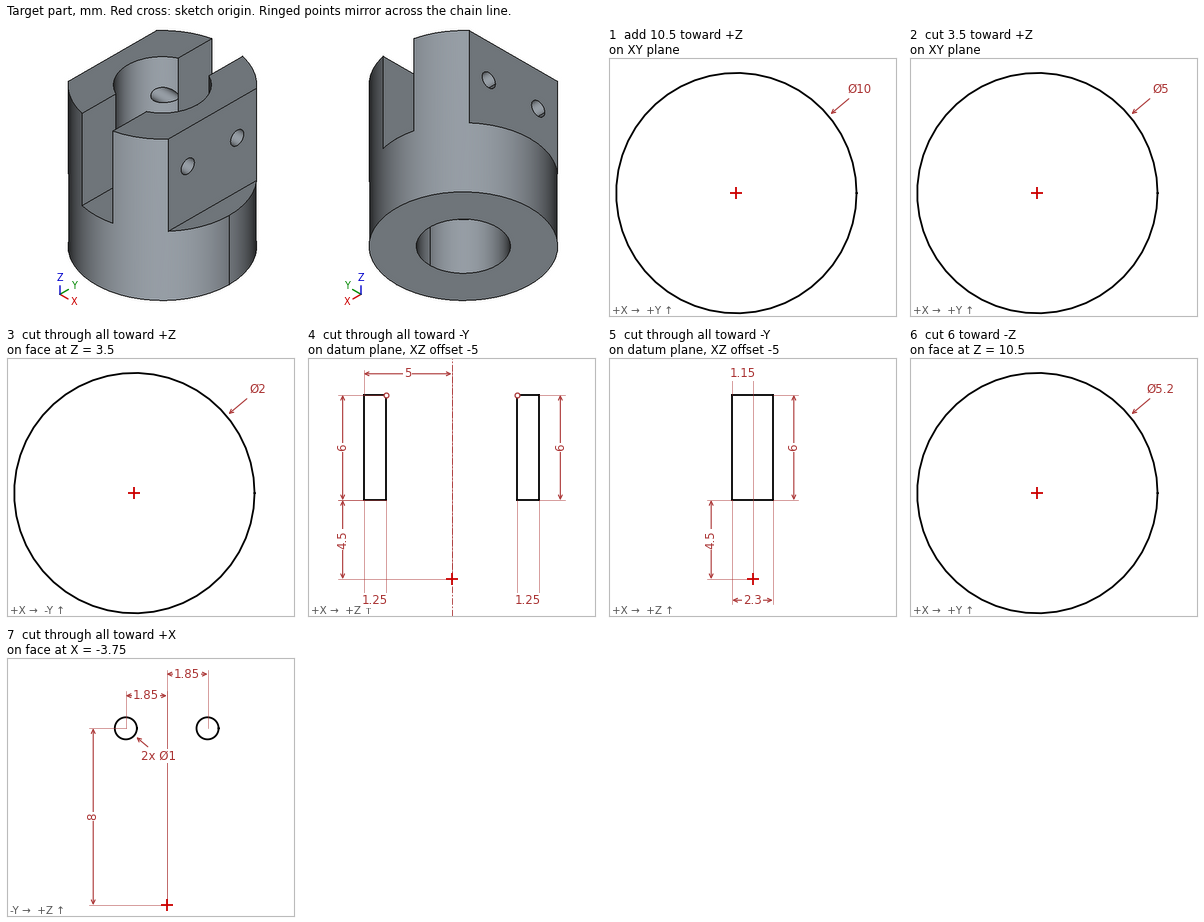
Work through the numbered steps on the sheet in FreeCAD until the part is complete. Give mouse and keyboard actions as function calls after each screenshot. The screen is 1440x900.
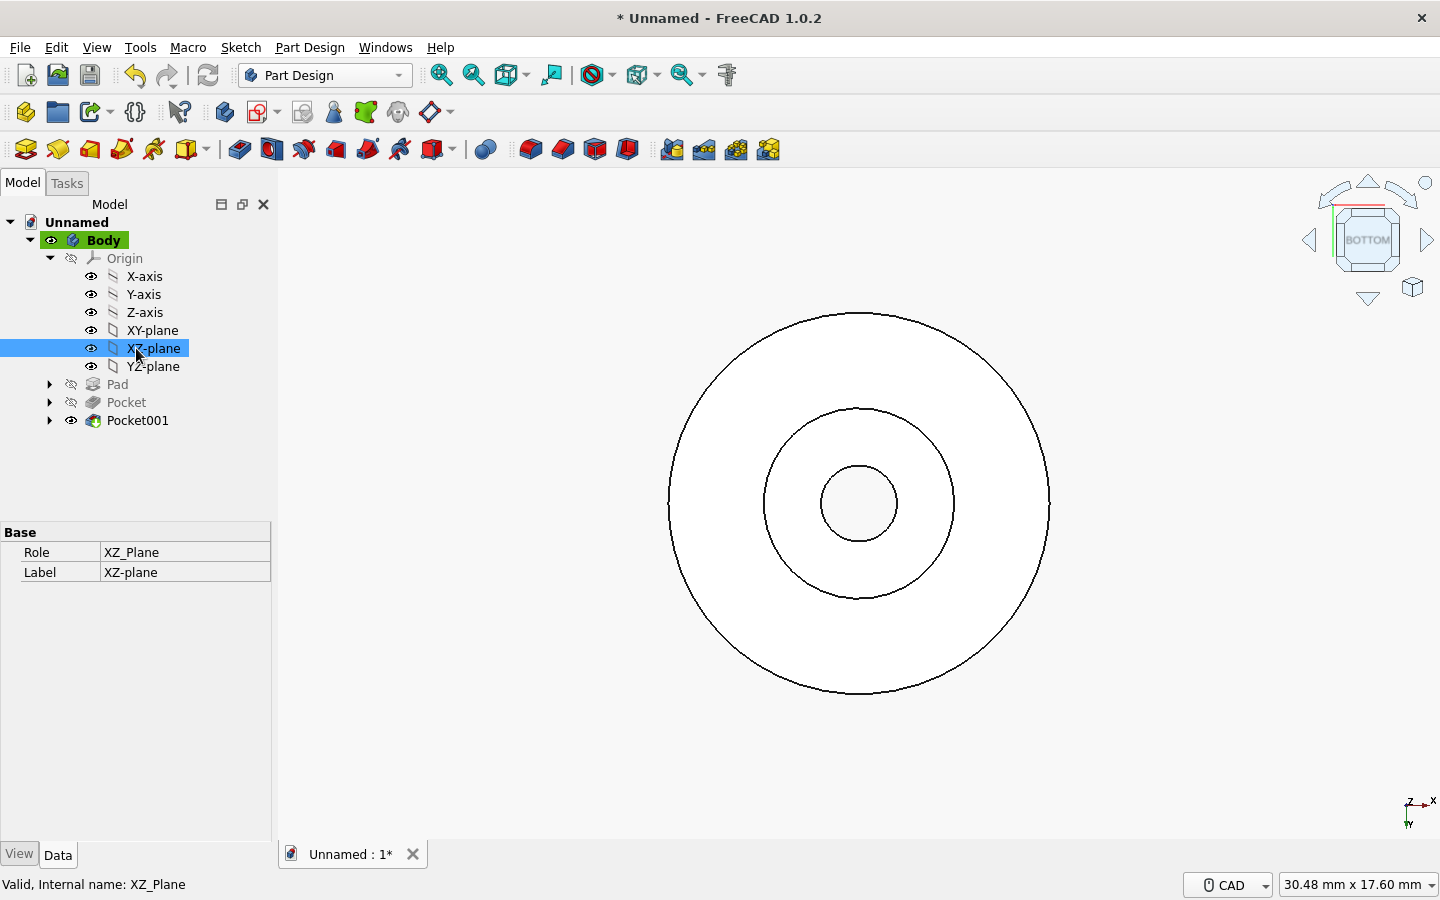
click(430, 112)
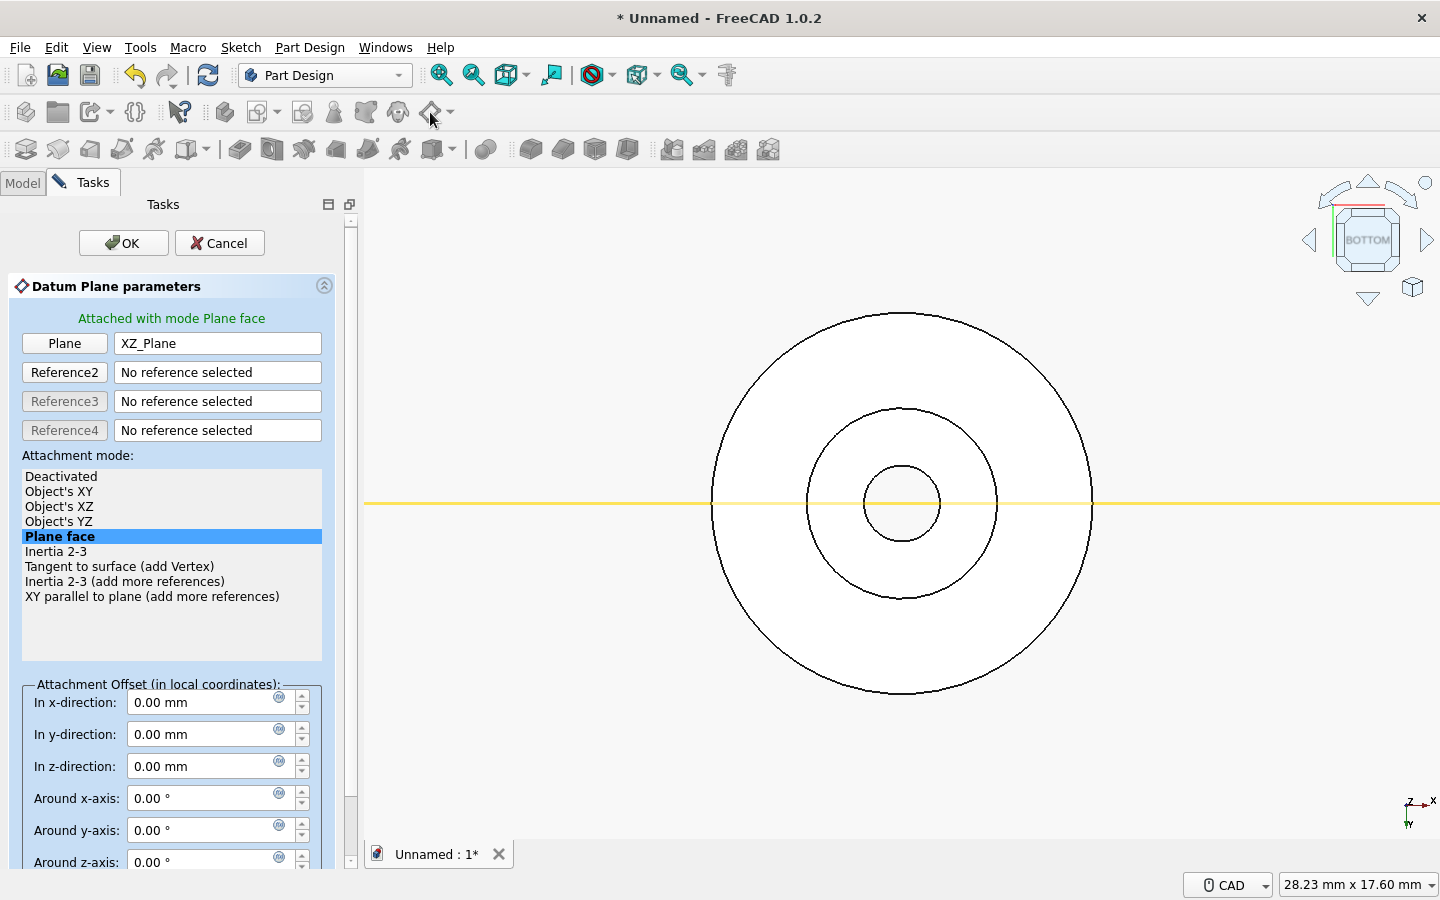
triple_click(210, 766)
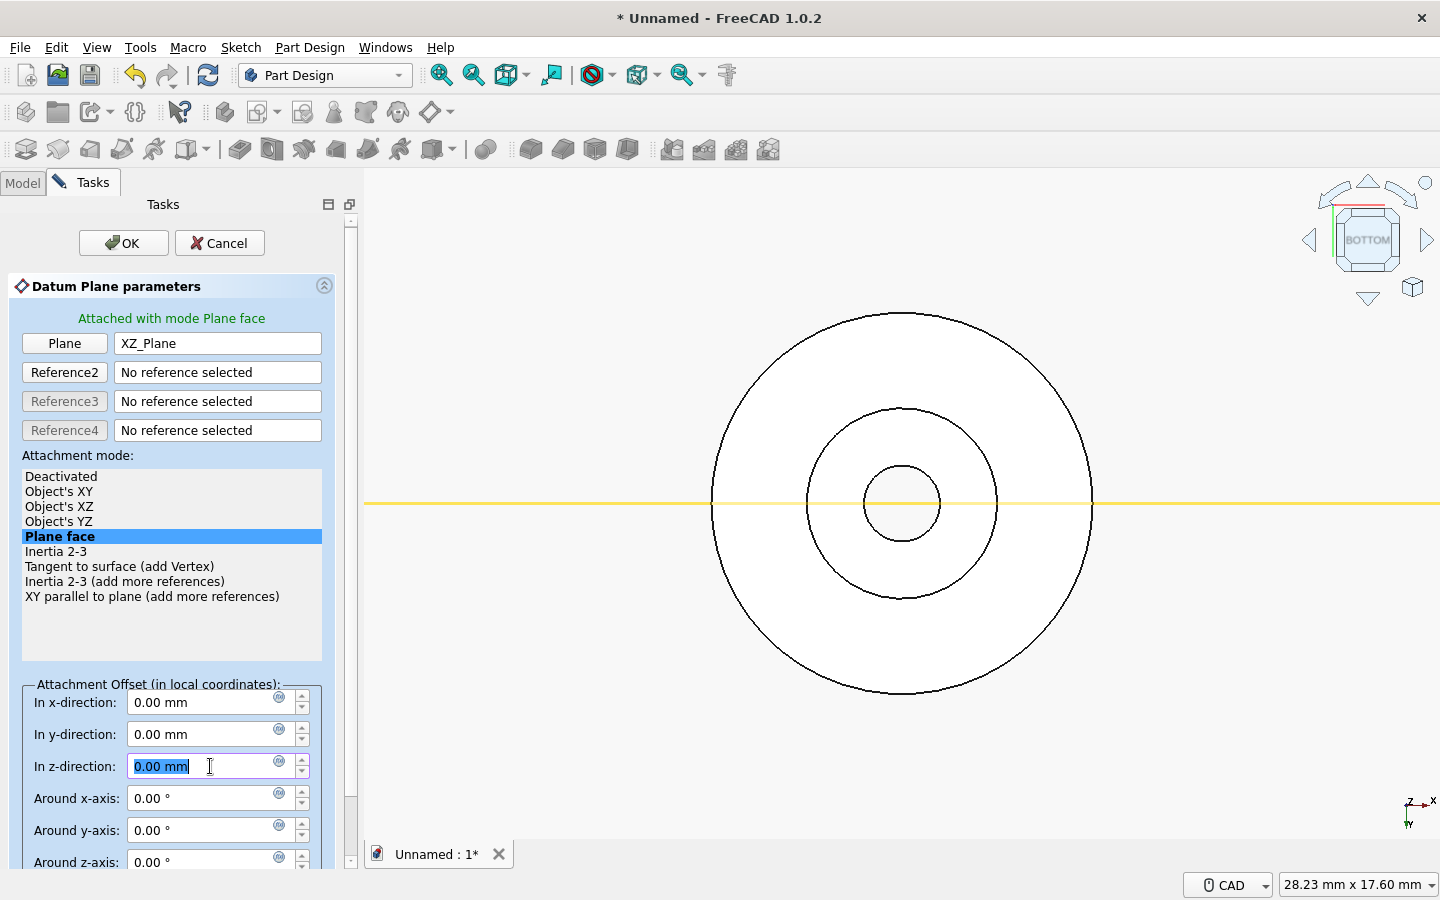
text(-5)
key(Tab)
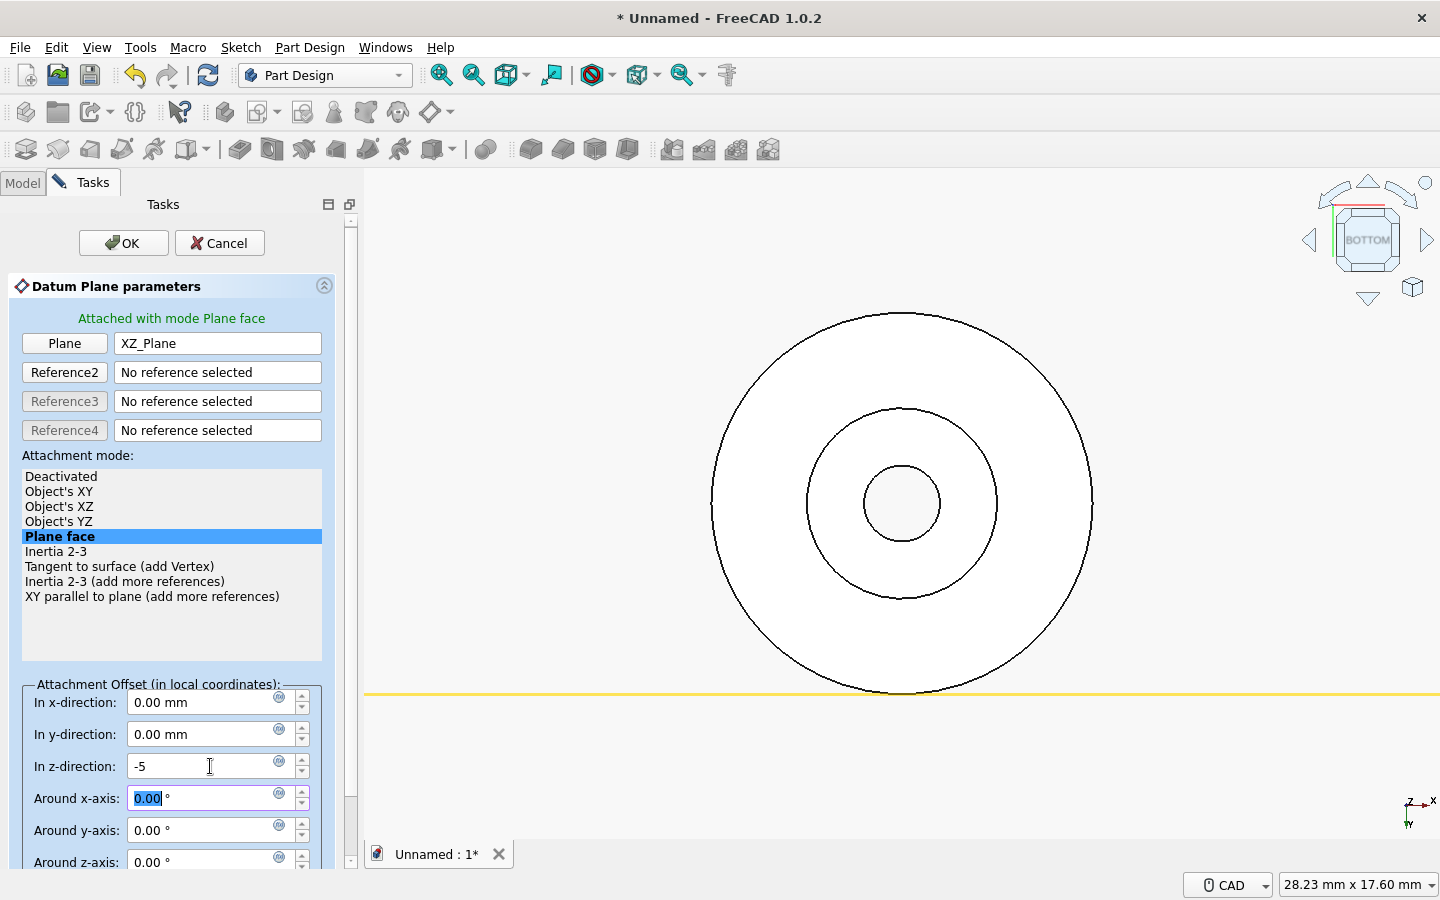
click(124, 243)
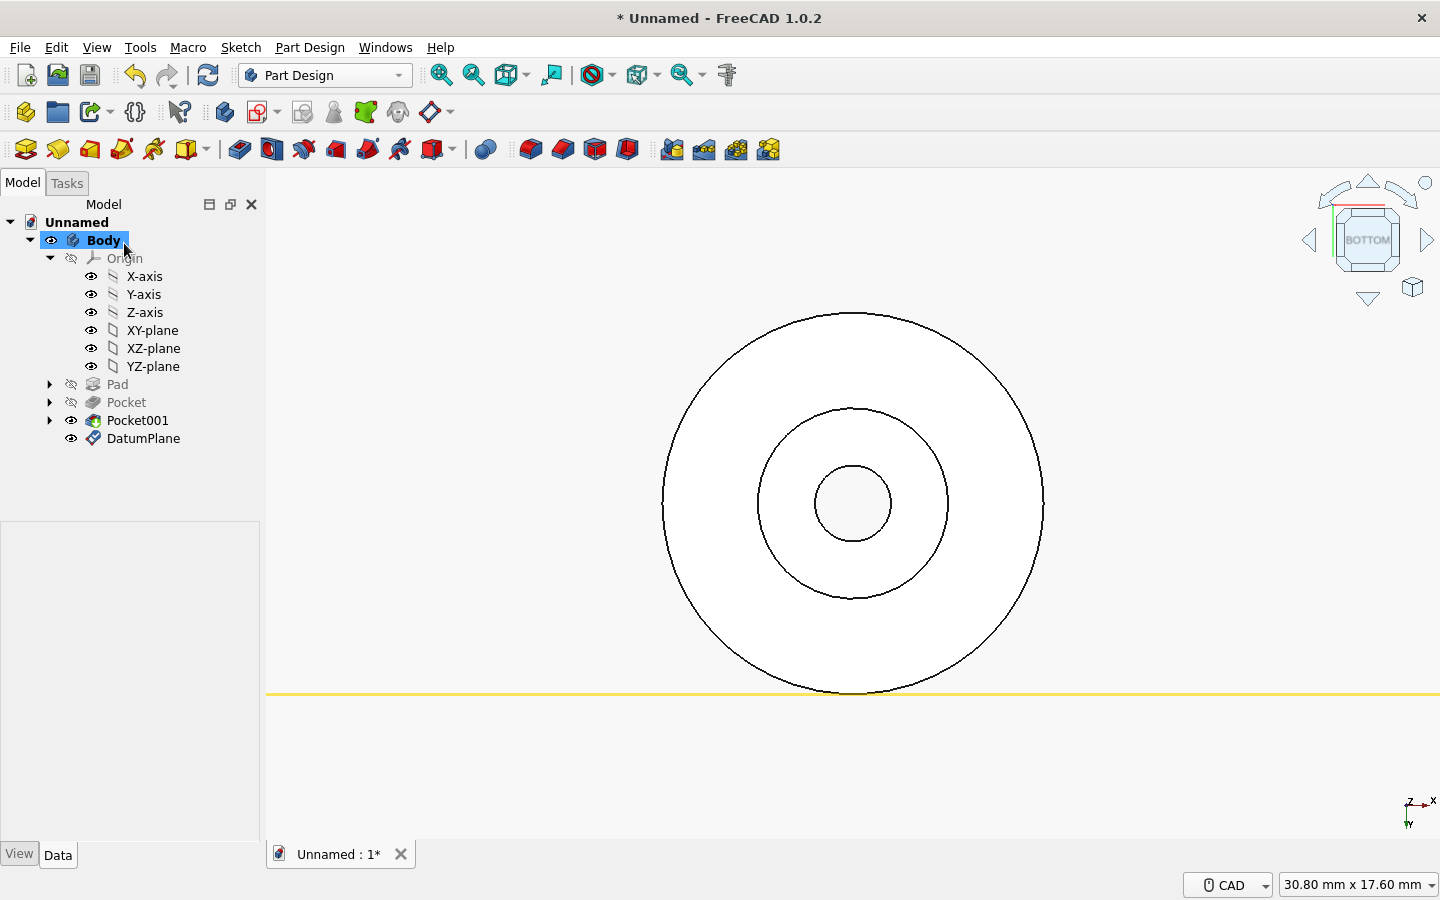
click(116, 438)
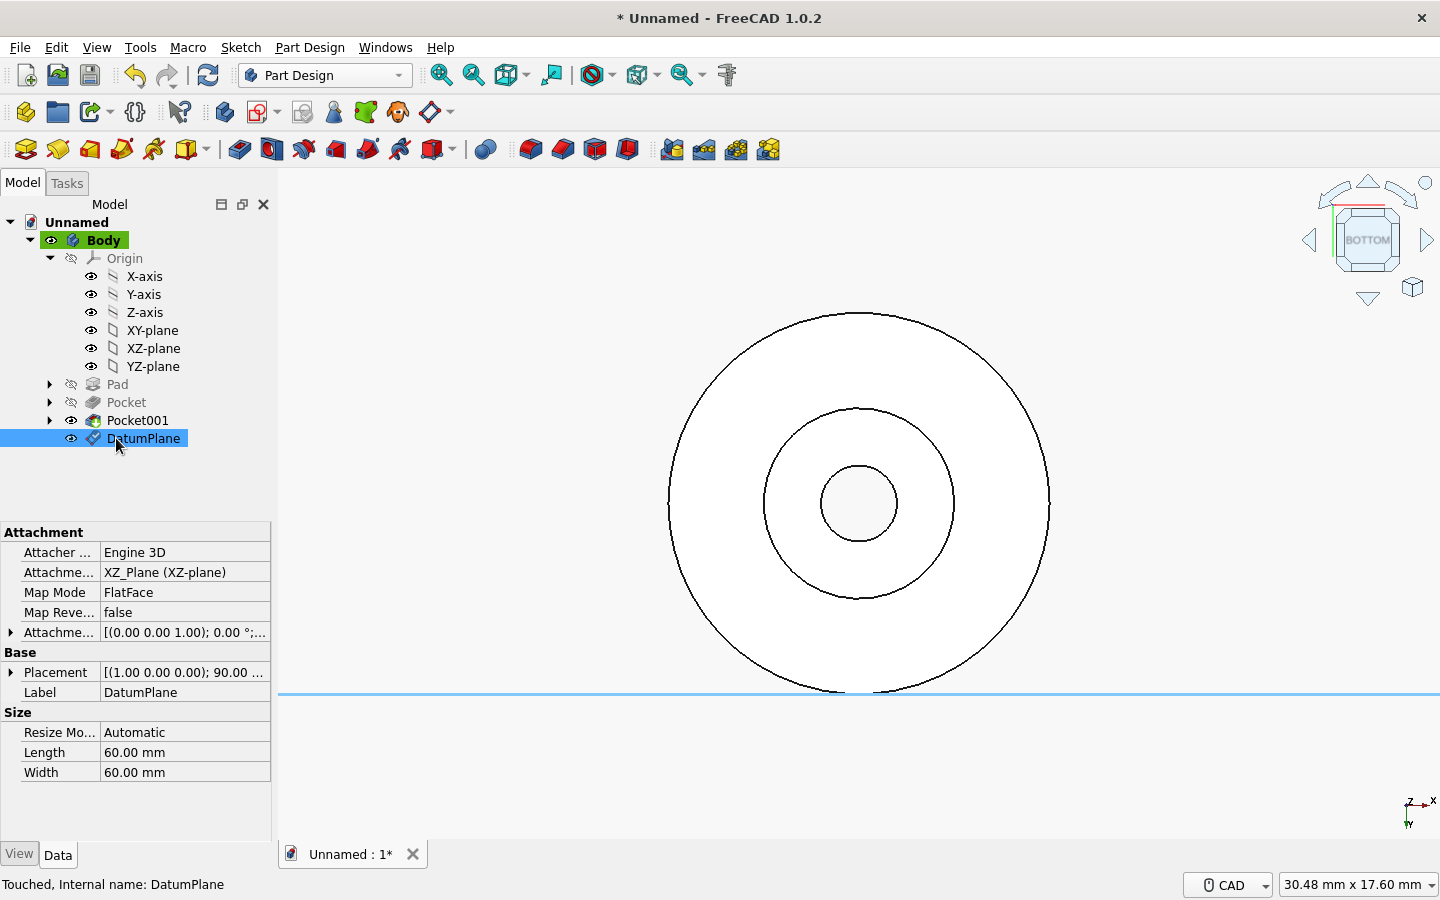
click(258, 112)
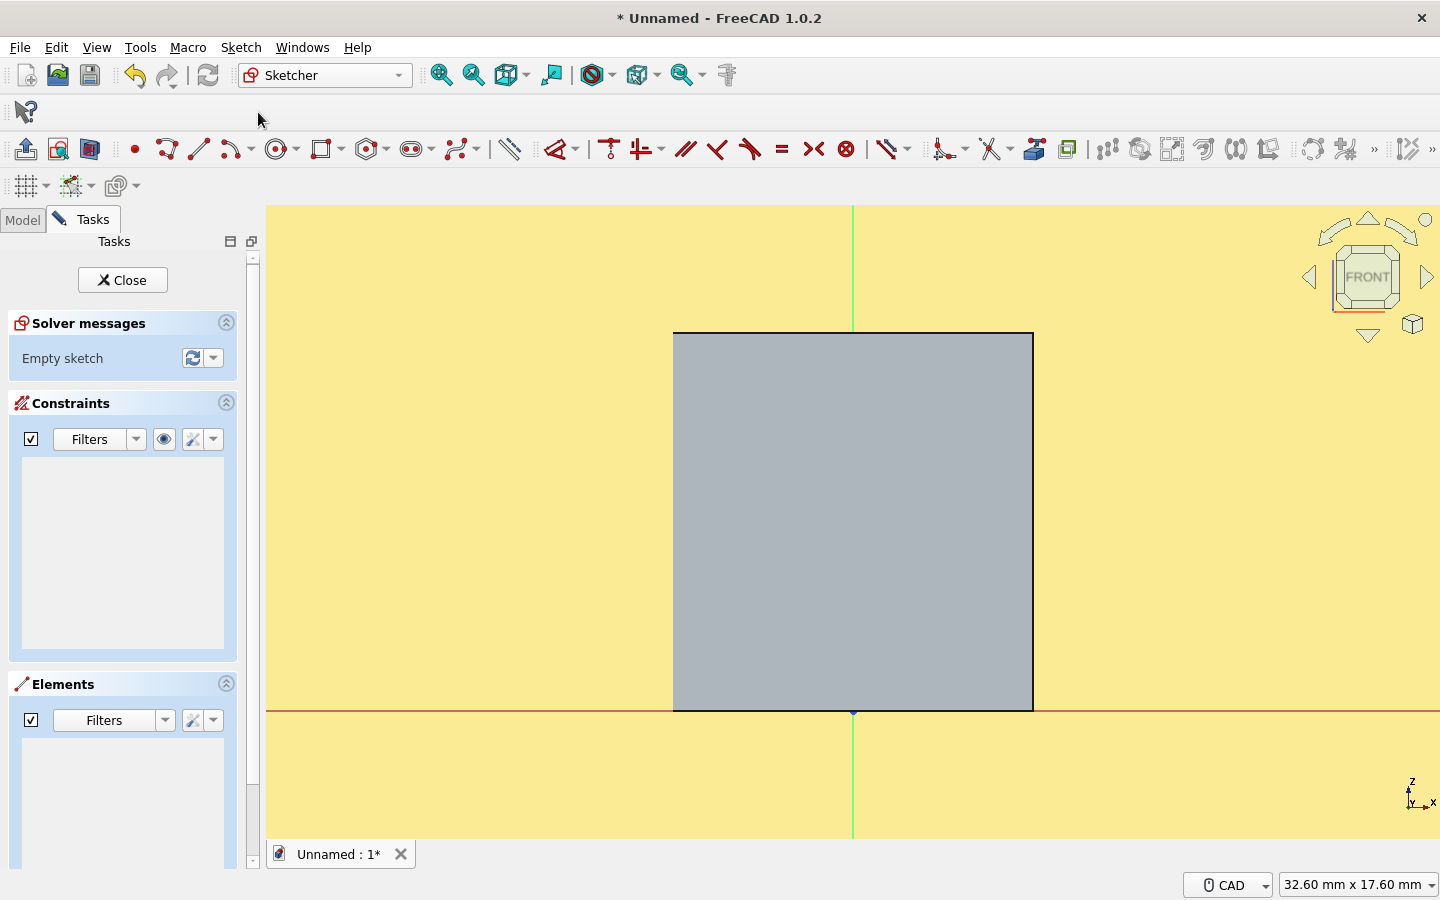
click(90, 150)